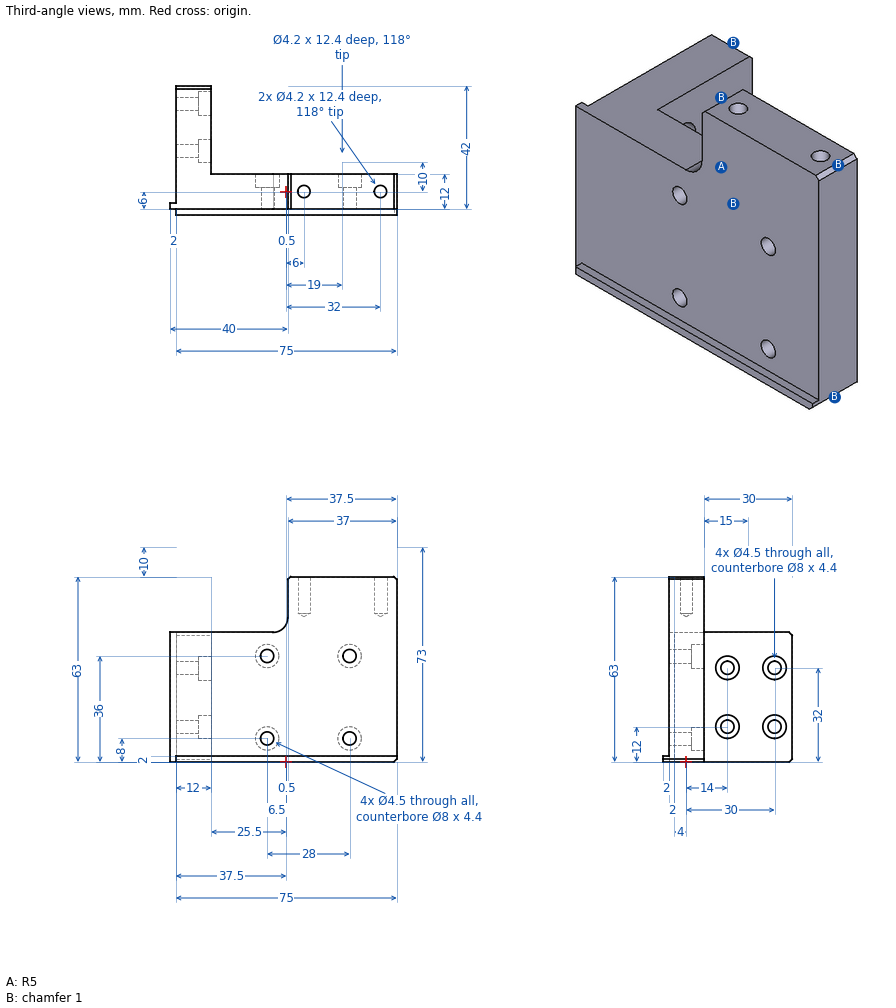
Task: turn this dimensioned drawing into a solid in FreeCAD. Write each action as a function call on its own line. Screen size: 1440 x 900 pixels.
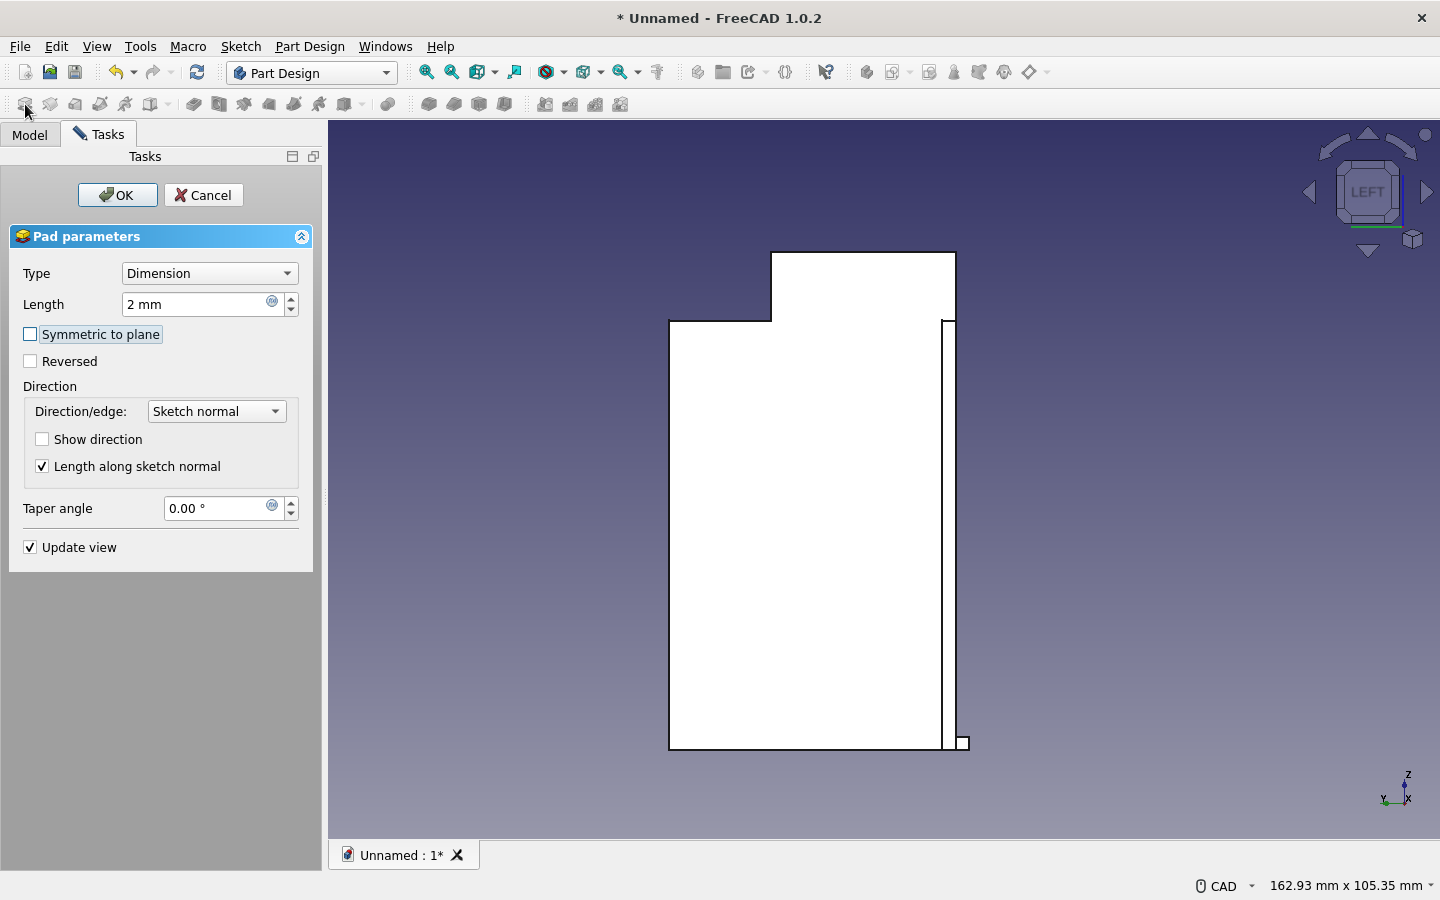
click(118, 195)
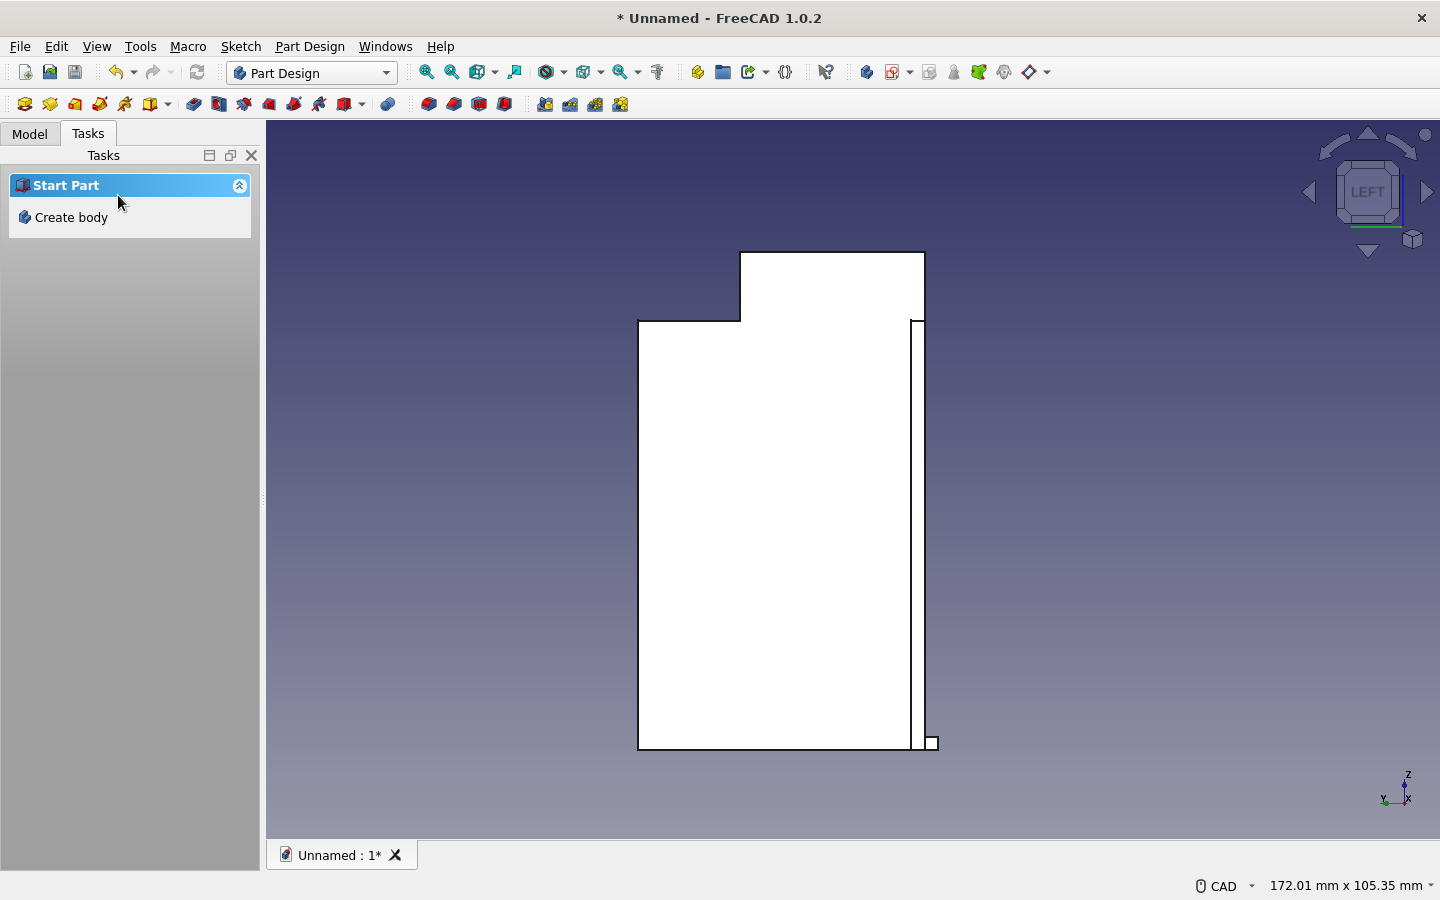
key(0)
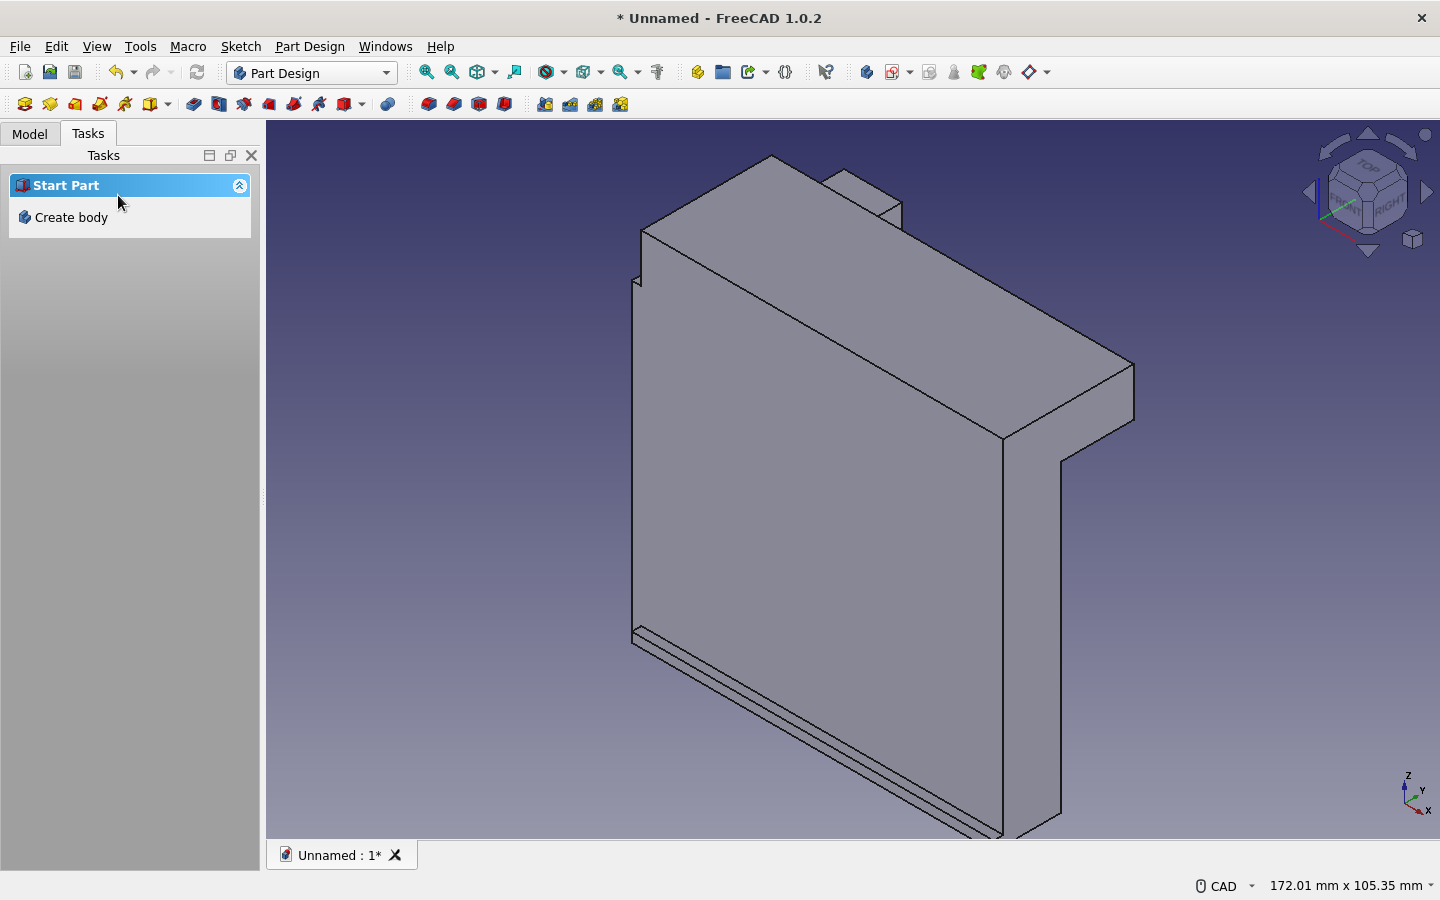
click(427, 72)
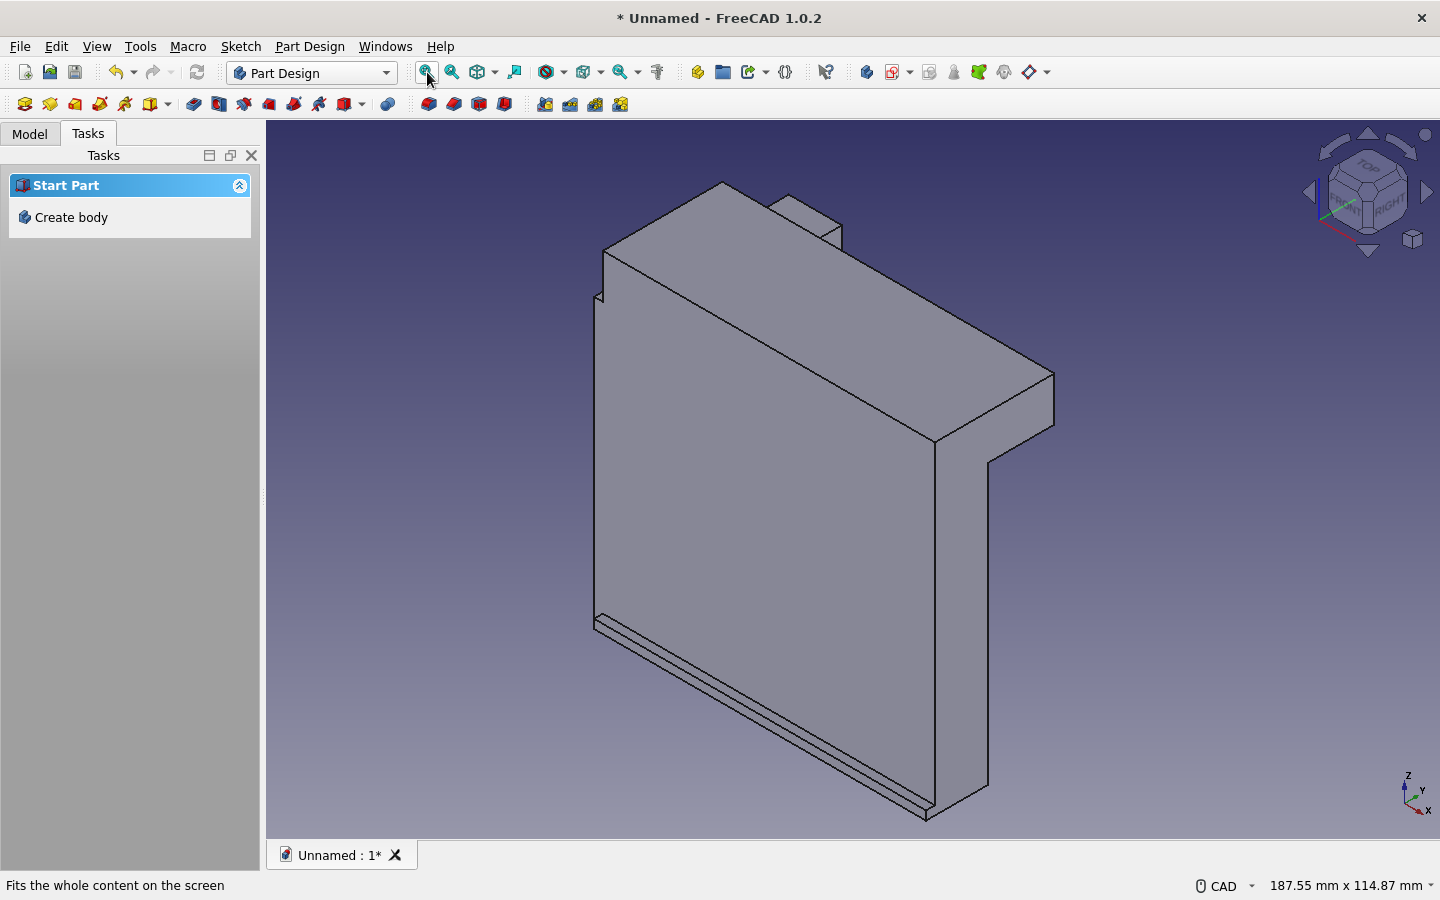
click(924, 366)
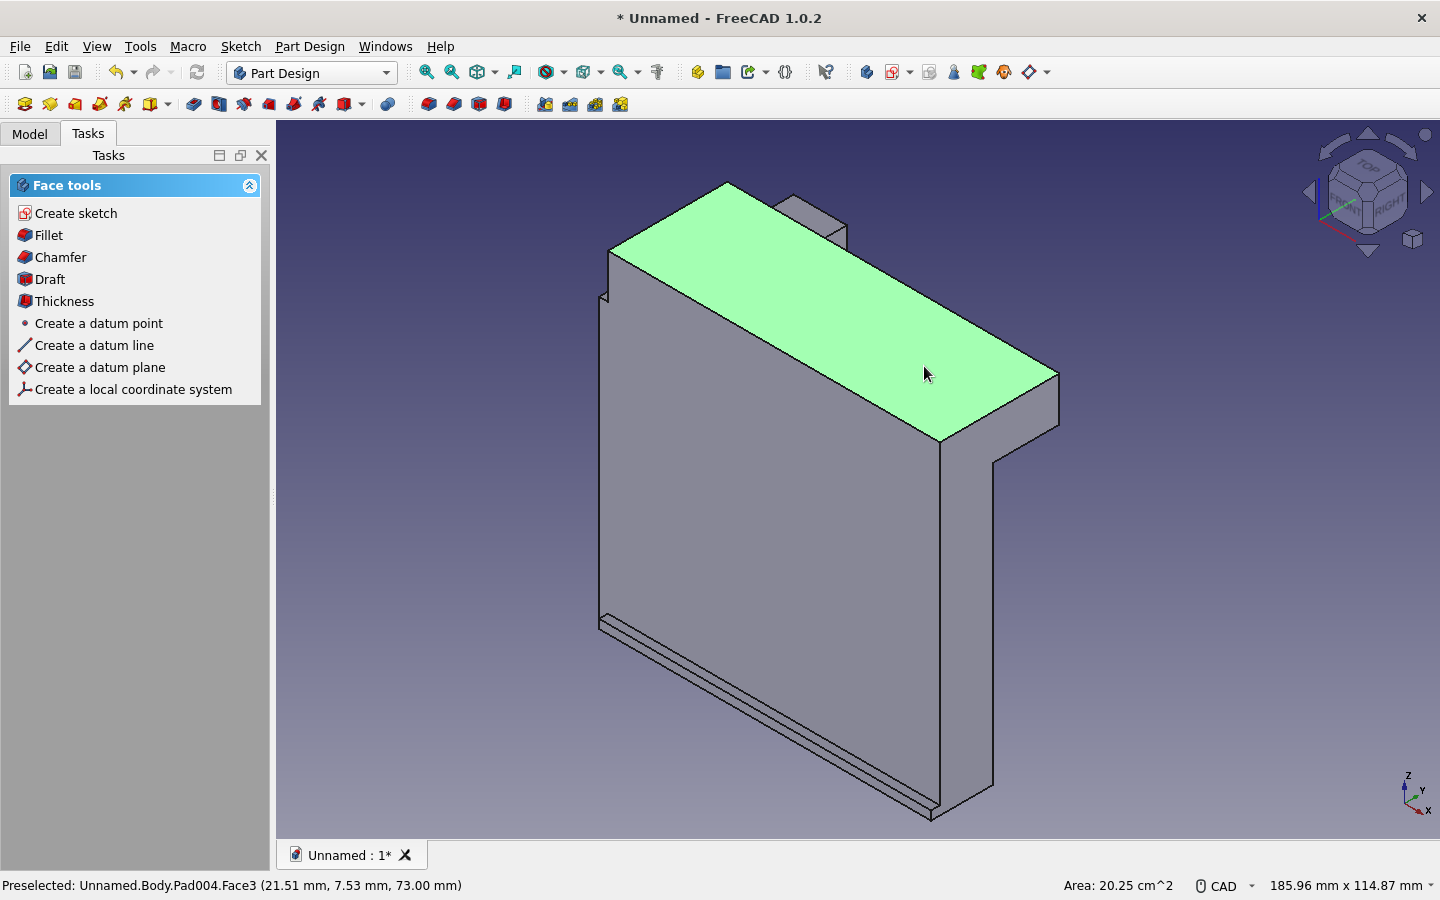
click(892, 72)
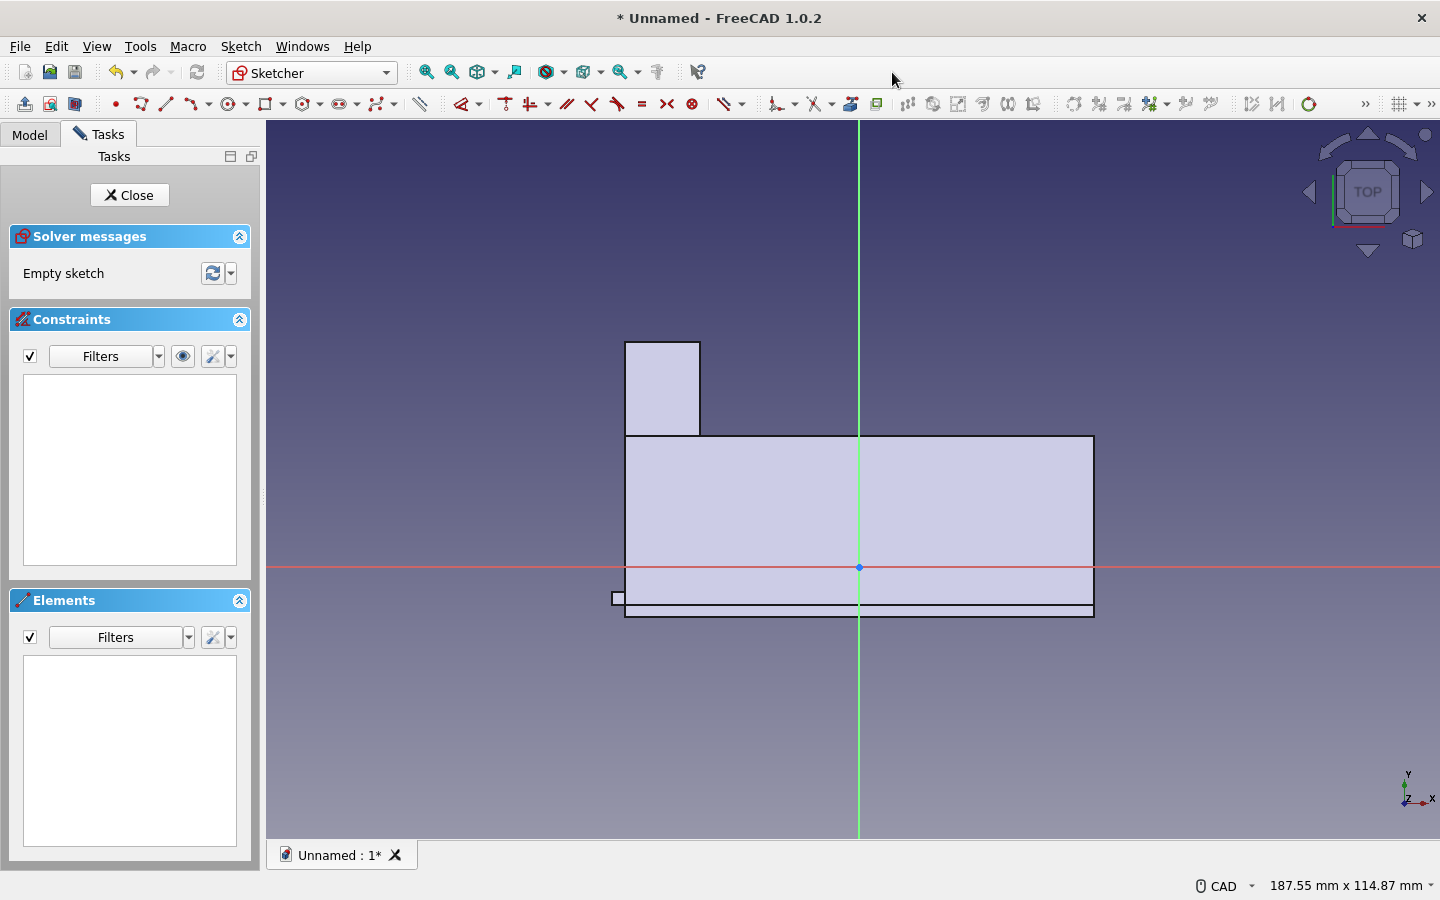
scroll(680, 466, up, 3)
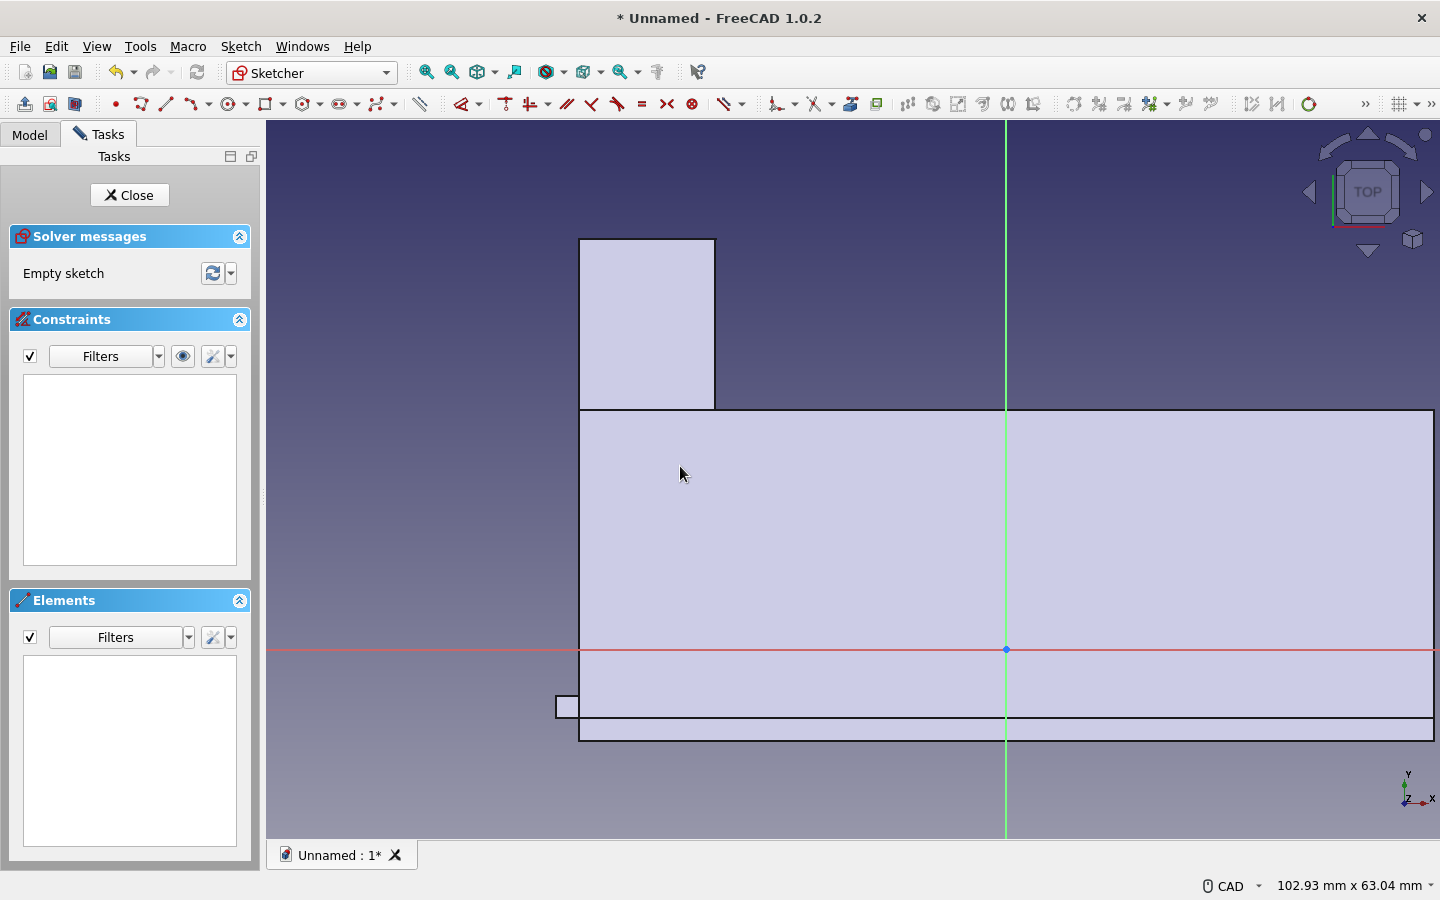
click(264, 104)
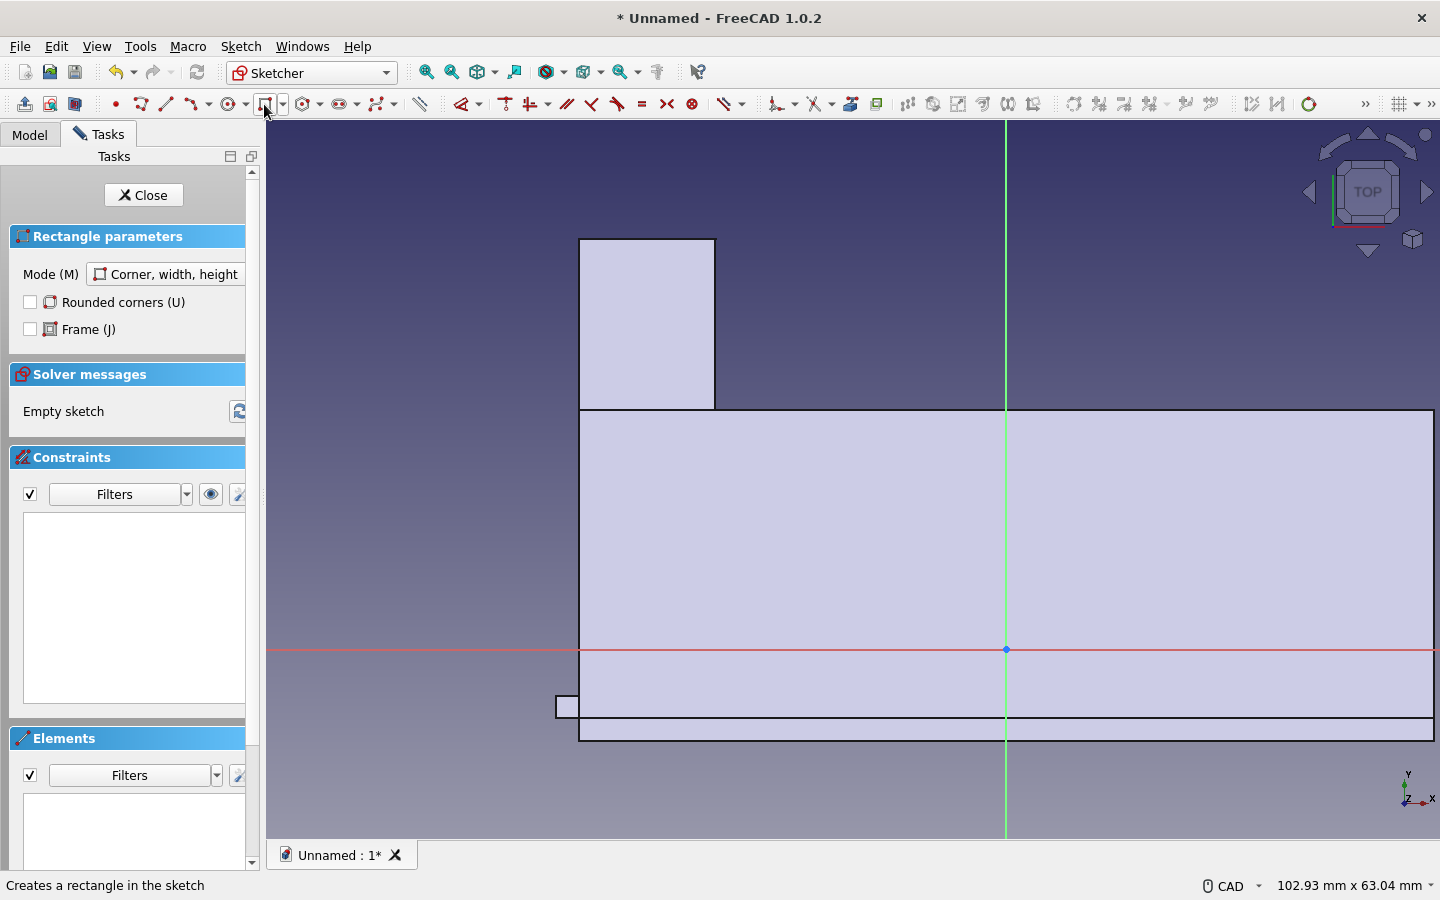
click(556, 239)